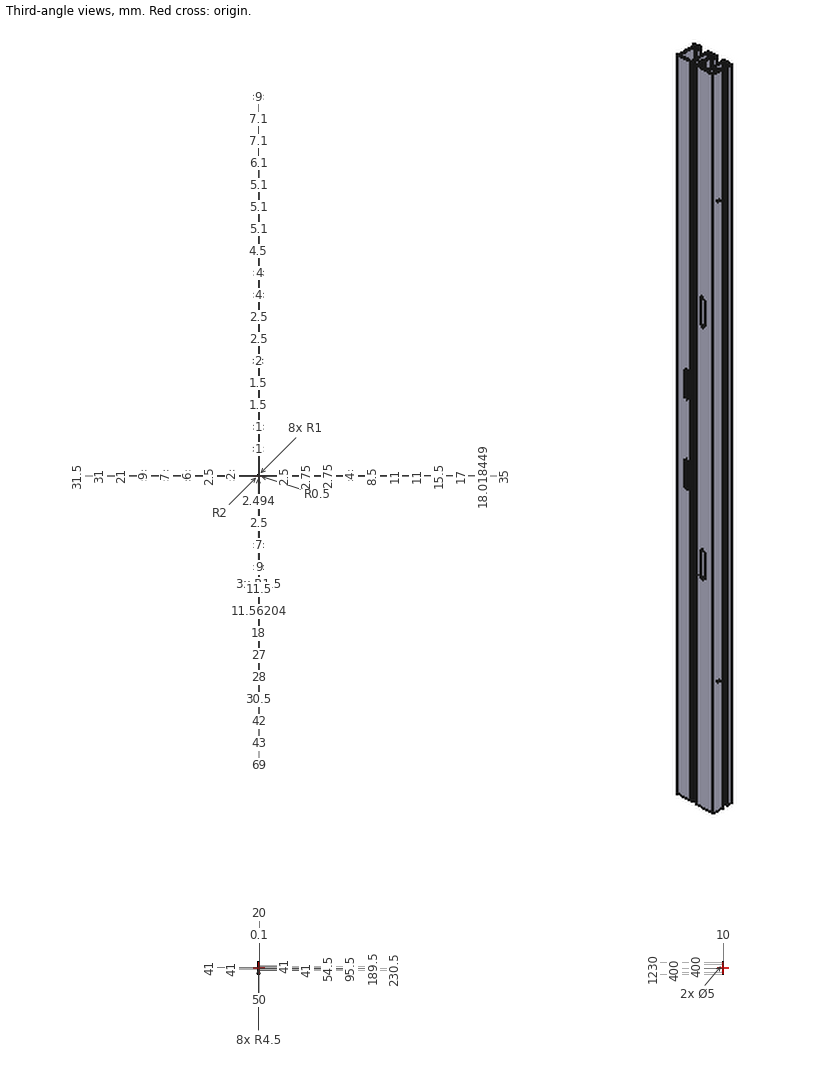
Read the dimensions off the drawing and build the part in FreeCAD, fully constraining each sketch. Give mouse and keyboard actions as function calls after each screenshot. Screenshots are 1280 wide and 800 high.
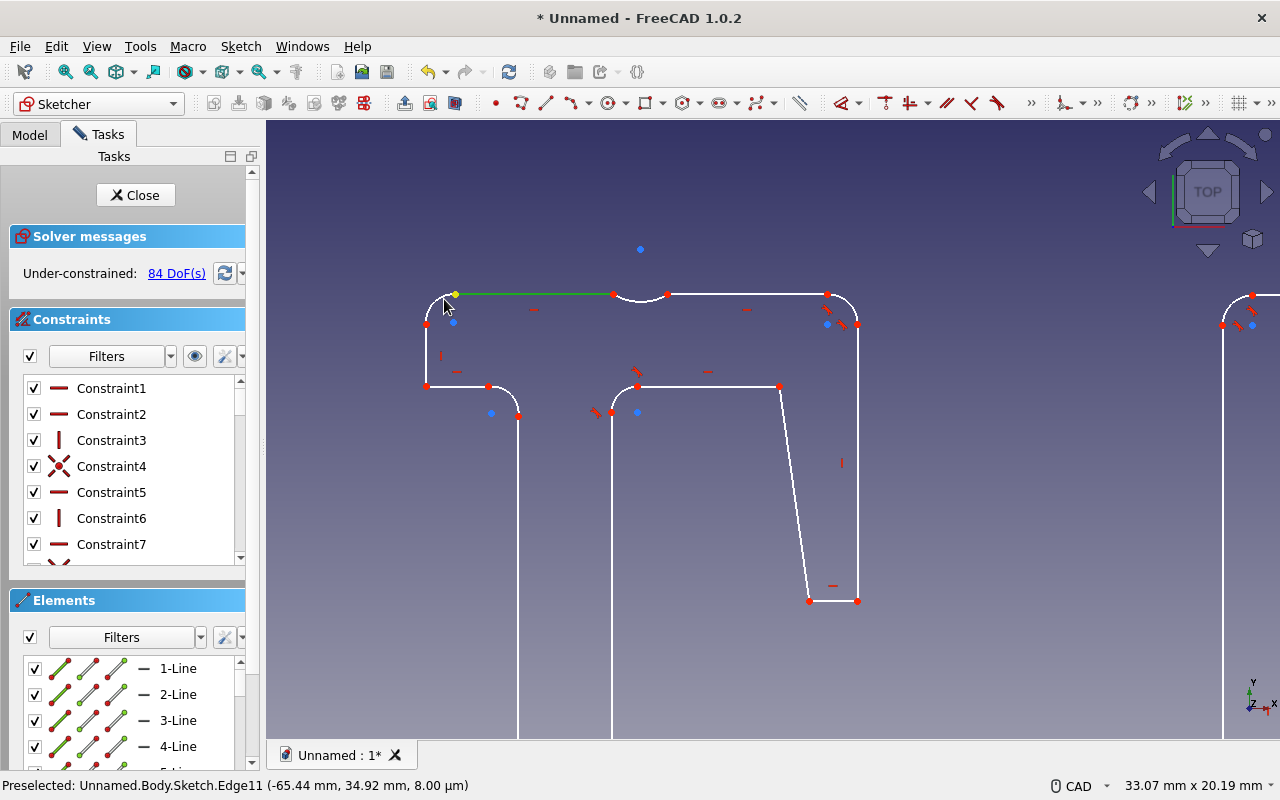
click(442, 297)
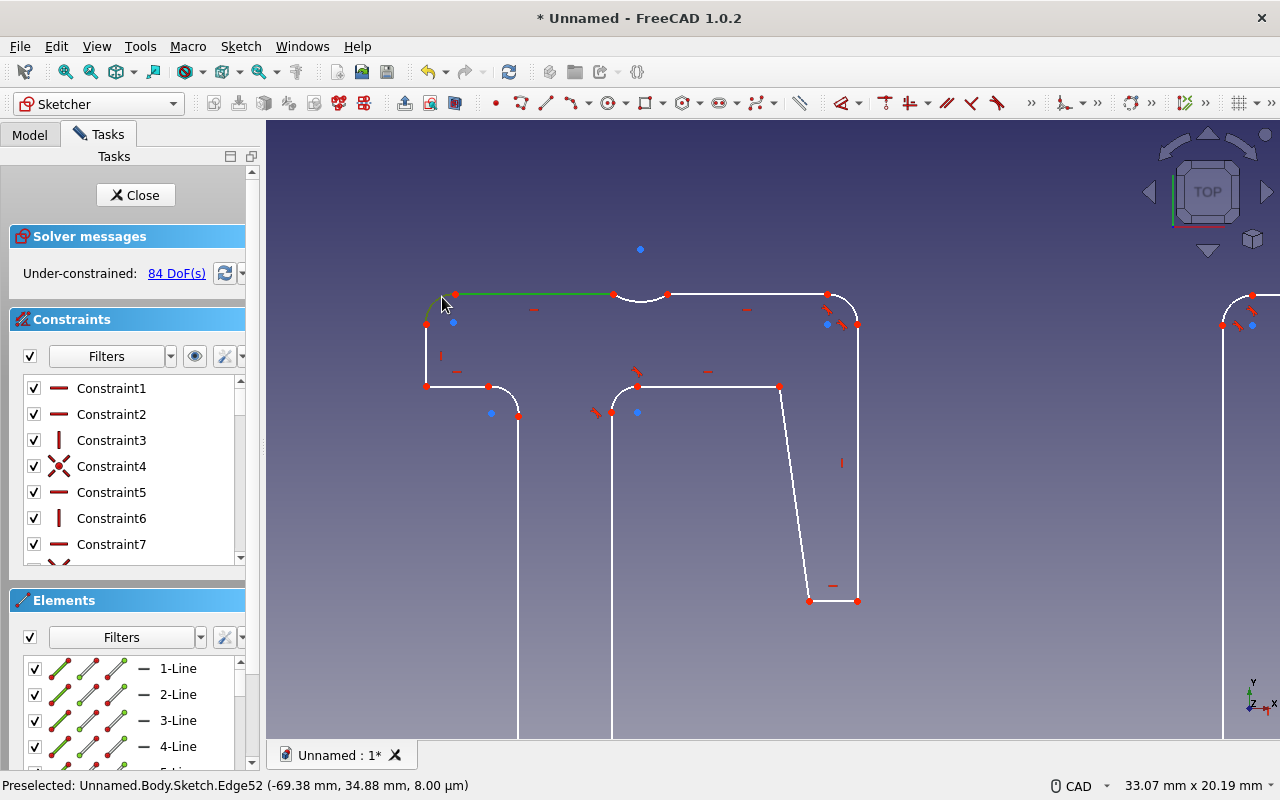
click(997, 104)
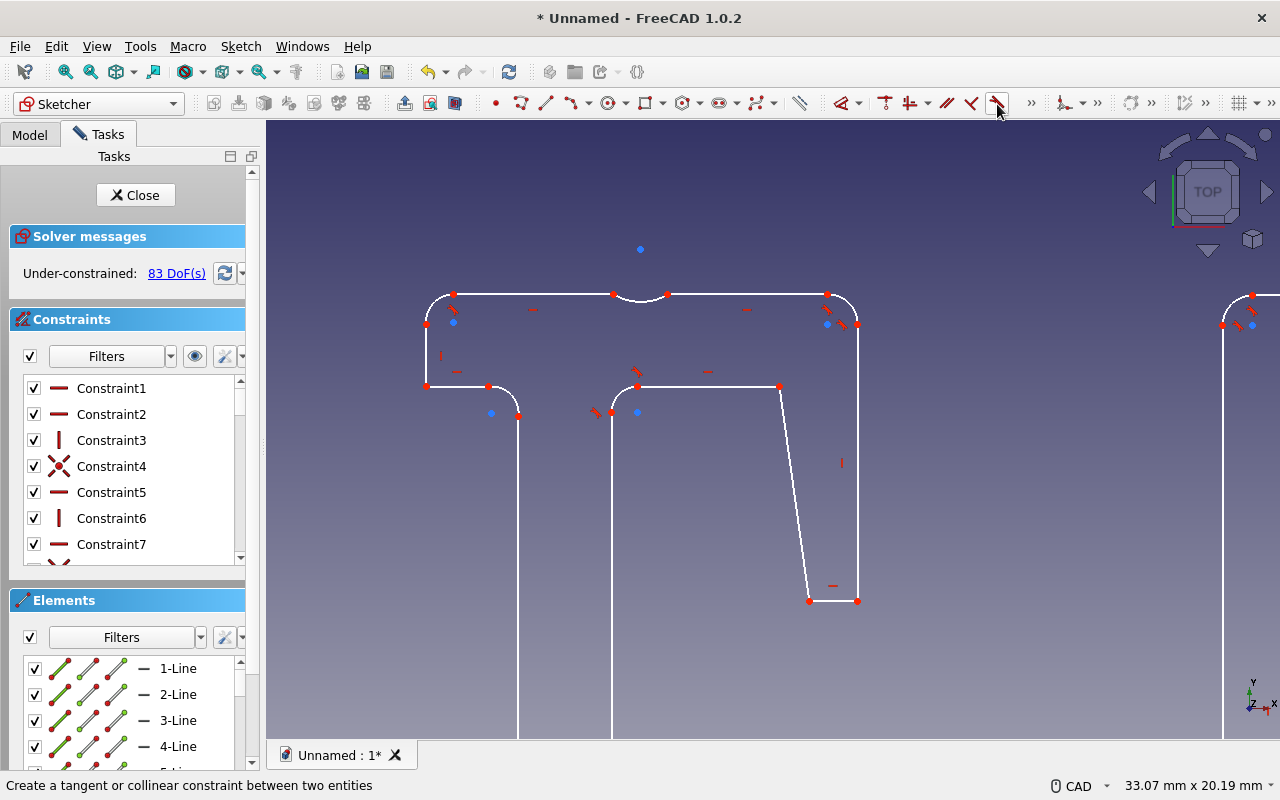
click(426, 343)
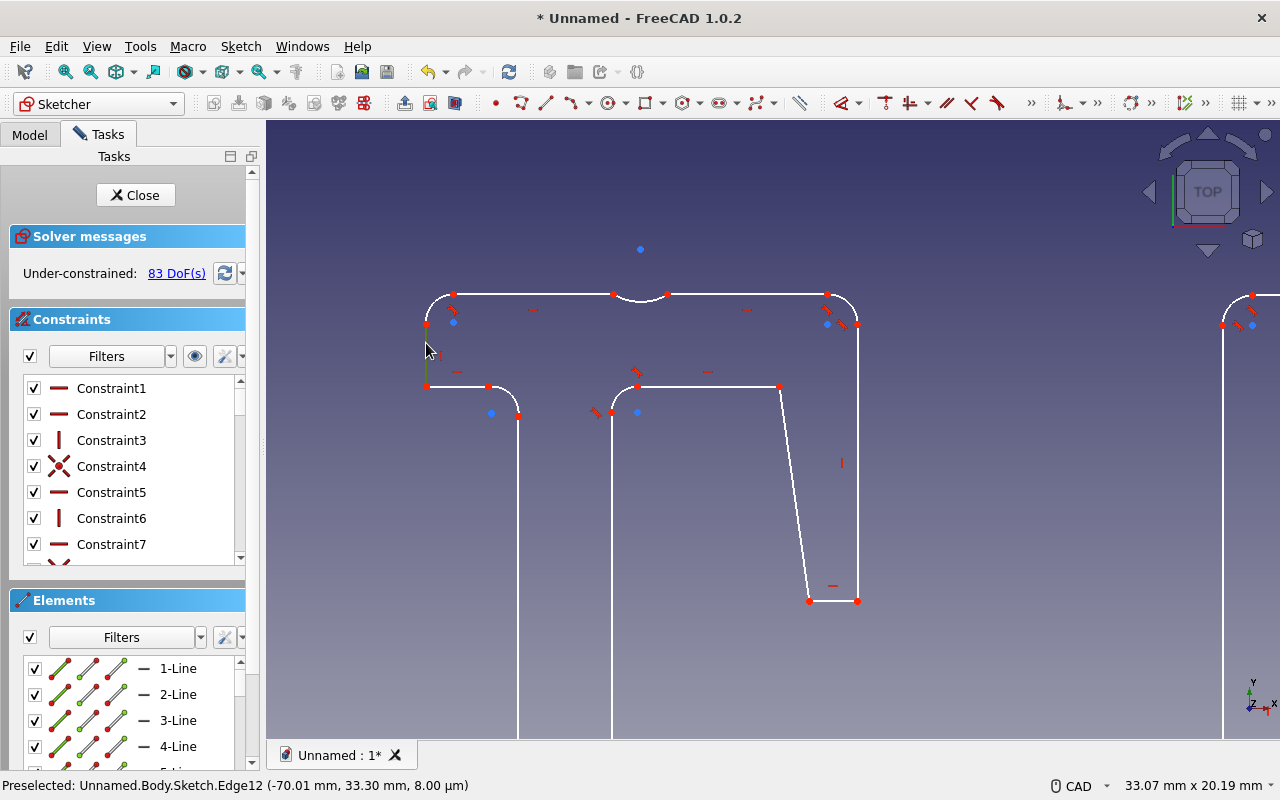
click(441, 298)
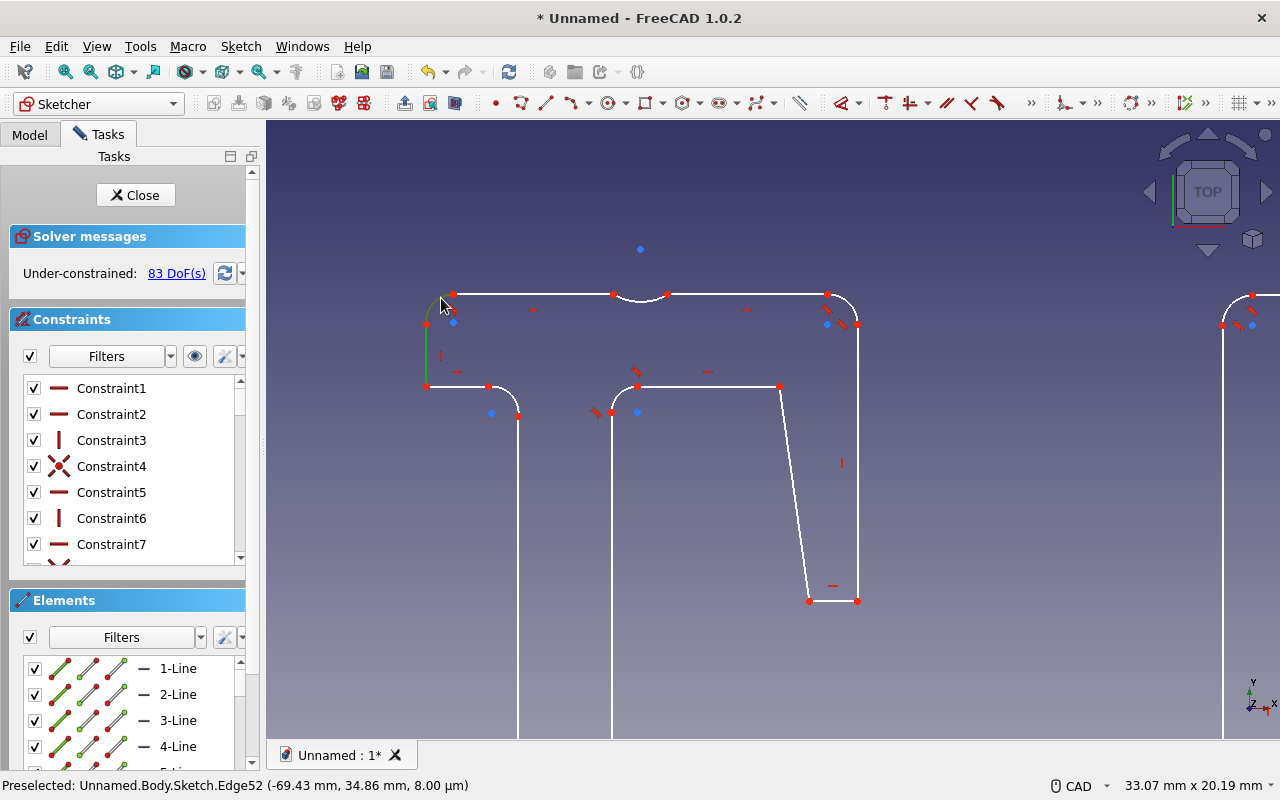
click(997, 104)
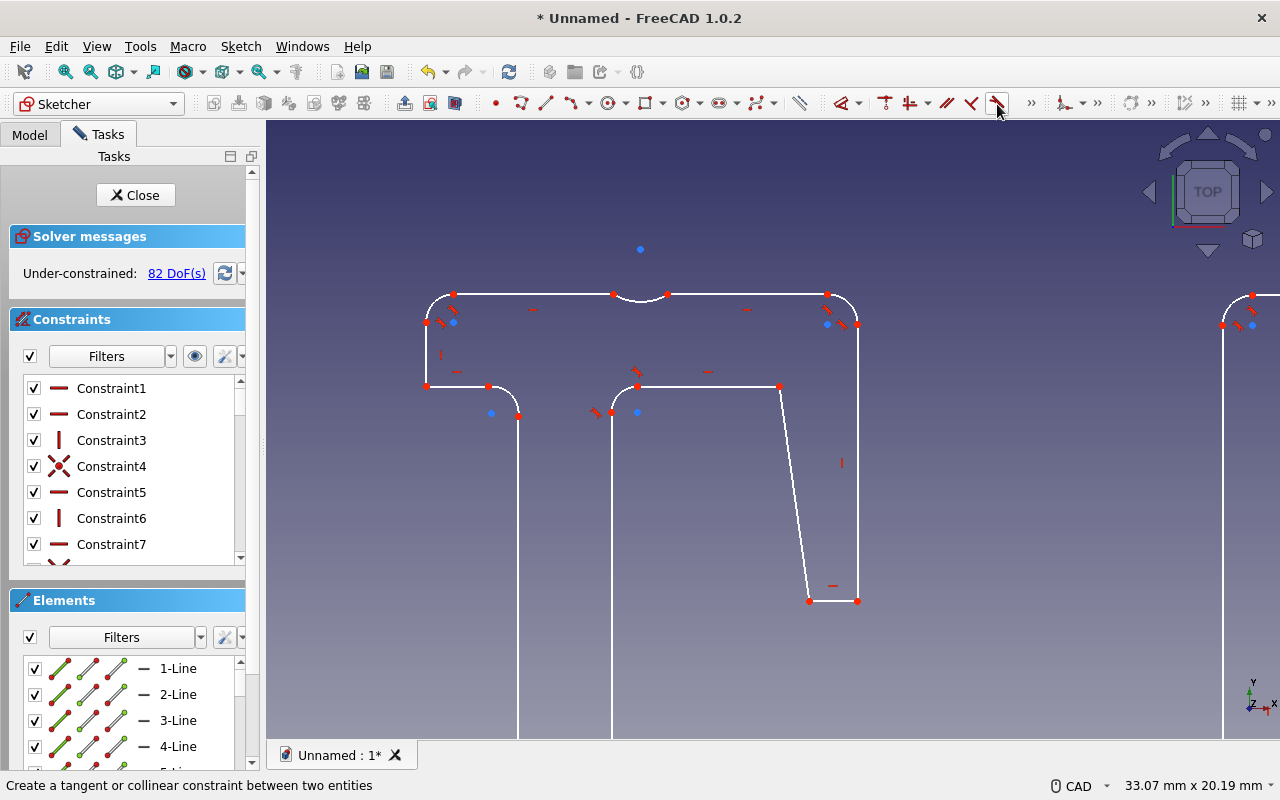
click(445, 387)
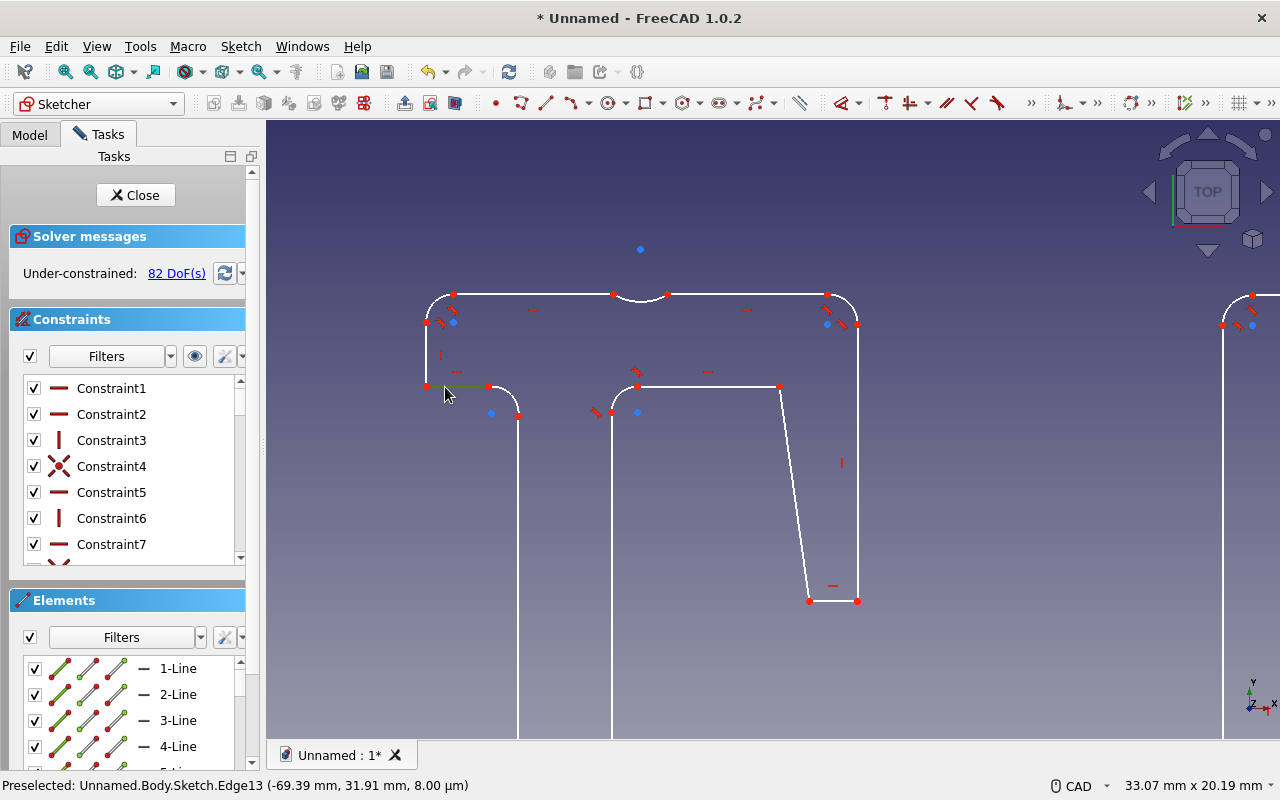
click(516, 402)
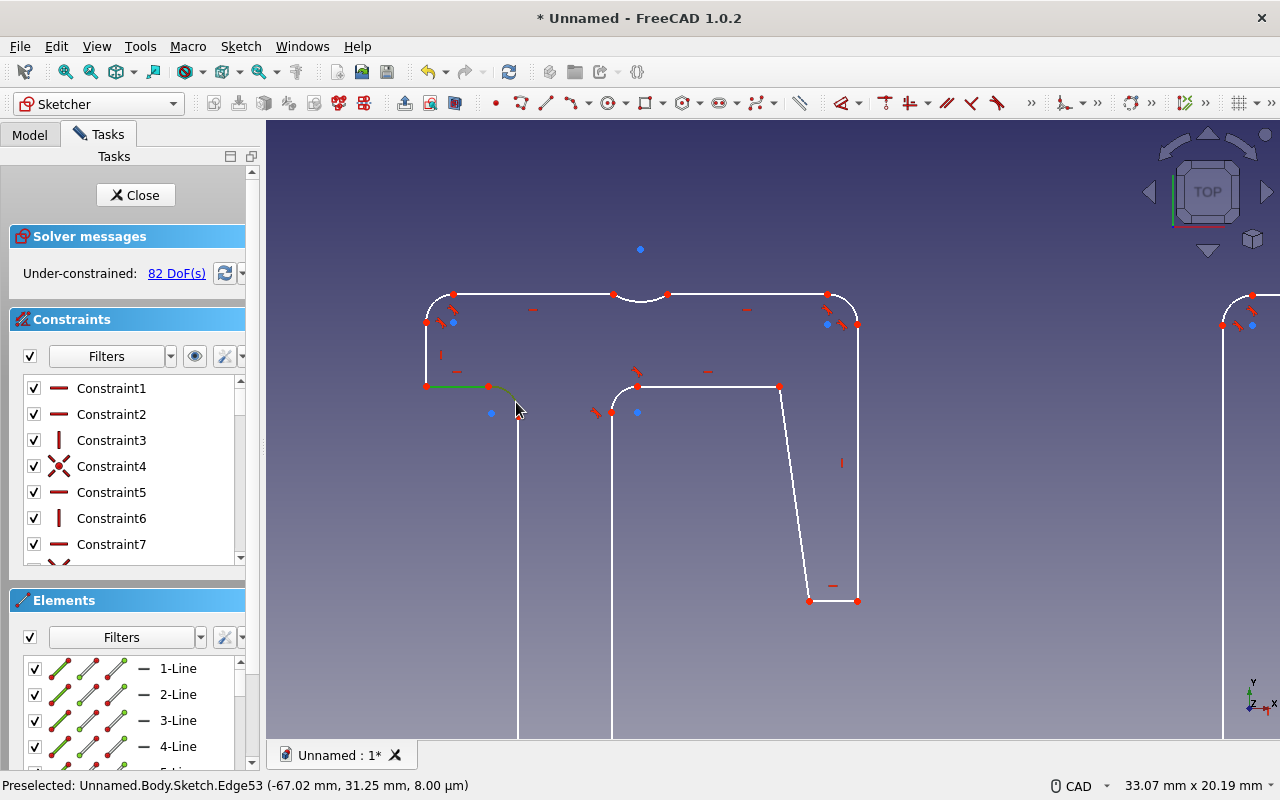
click(997, 104)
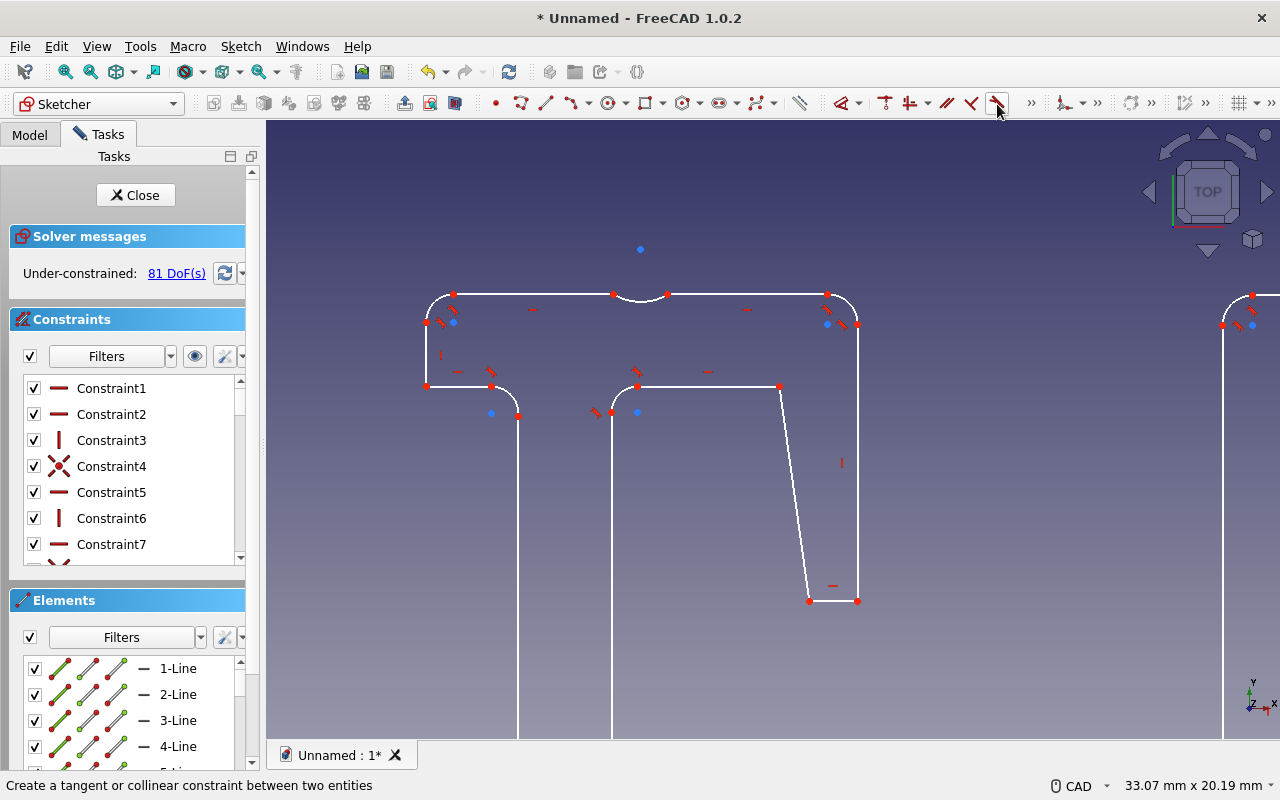
scroll(444, 299, down, 7)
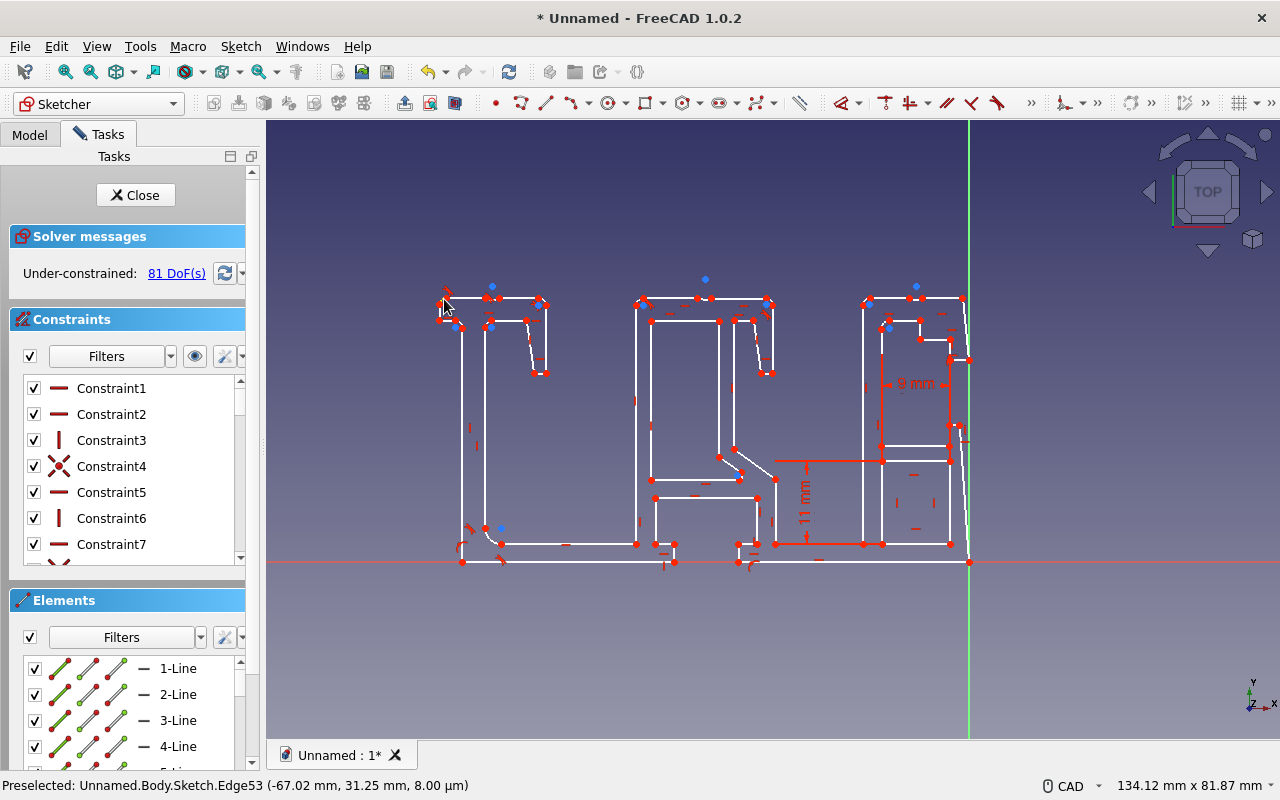
click(462, 398)